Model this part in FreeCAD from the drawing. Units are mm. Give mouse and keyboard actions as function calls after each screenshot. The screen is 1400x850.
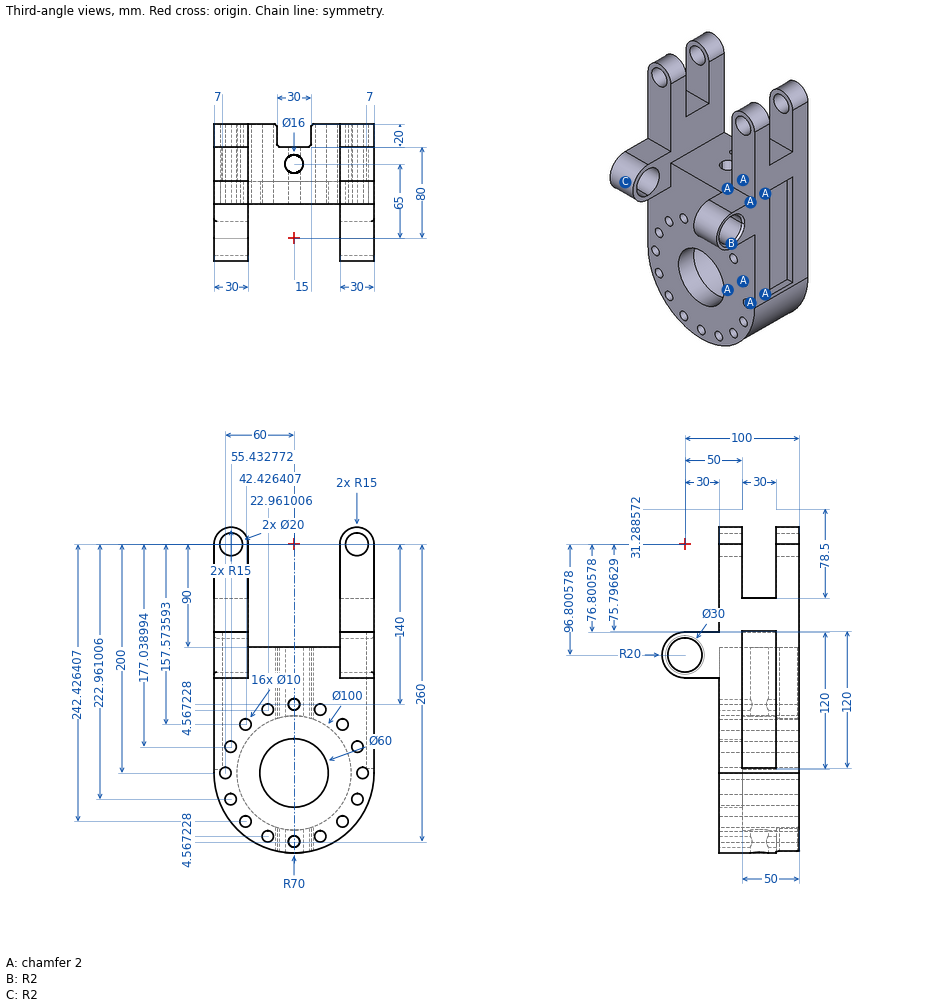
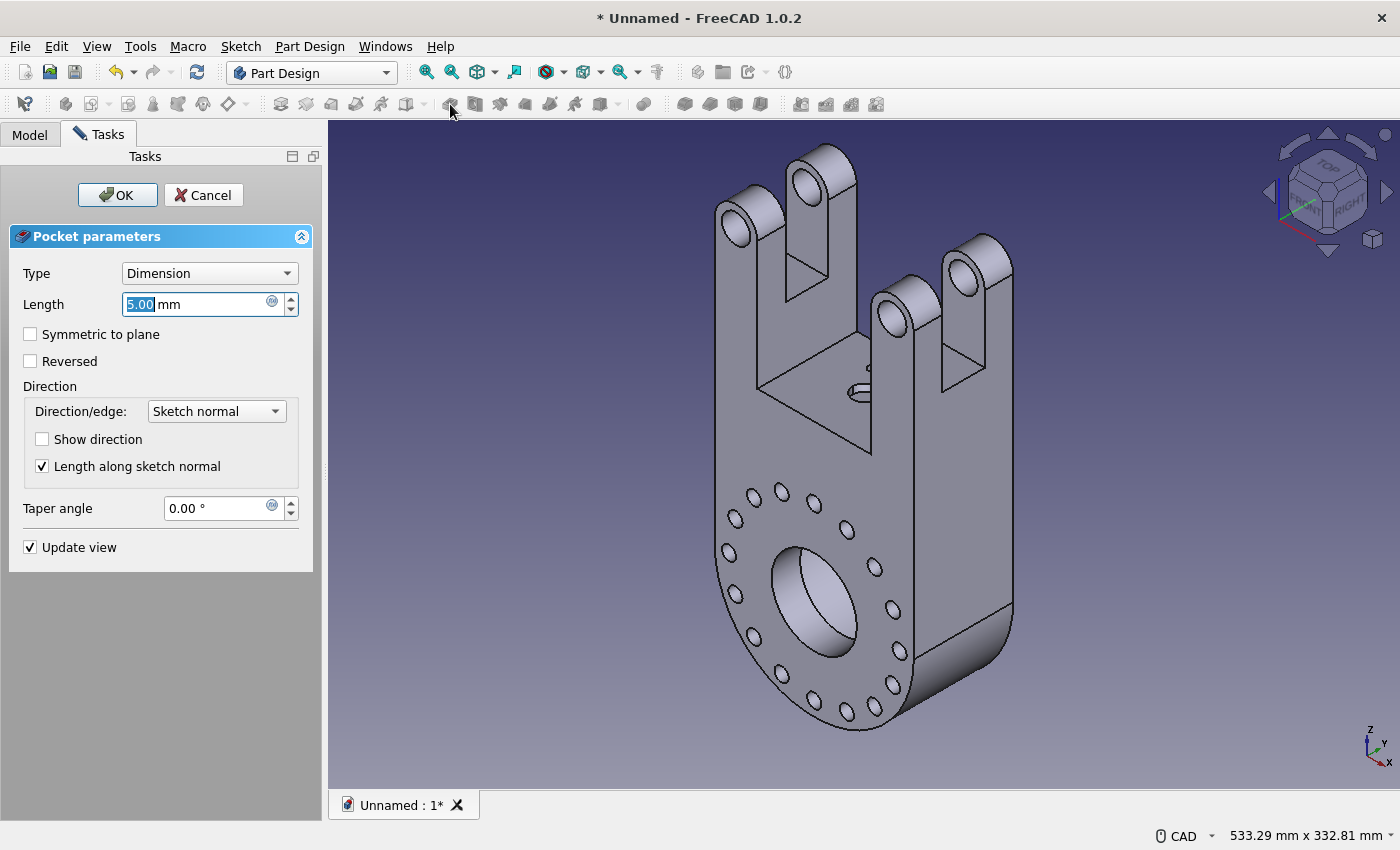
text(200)
key(Tab)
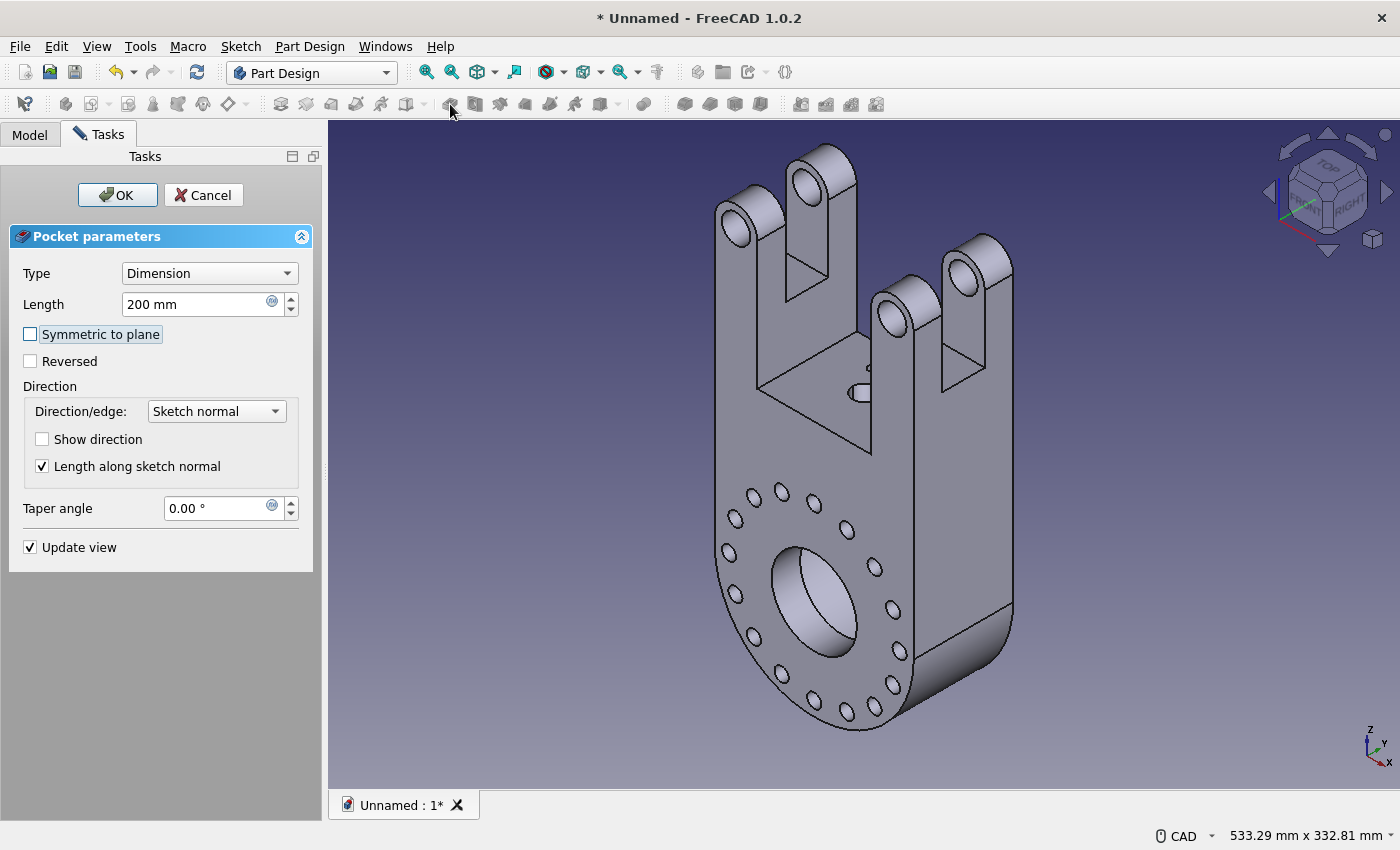
click(118, 195)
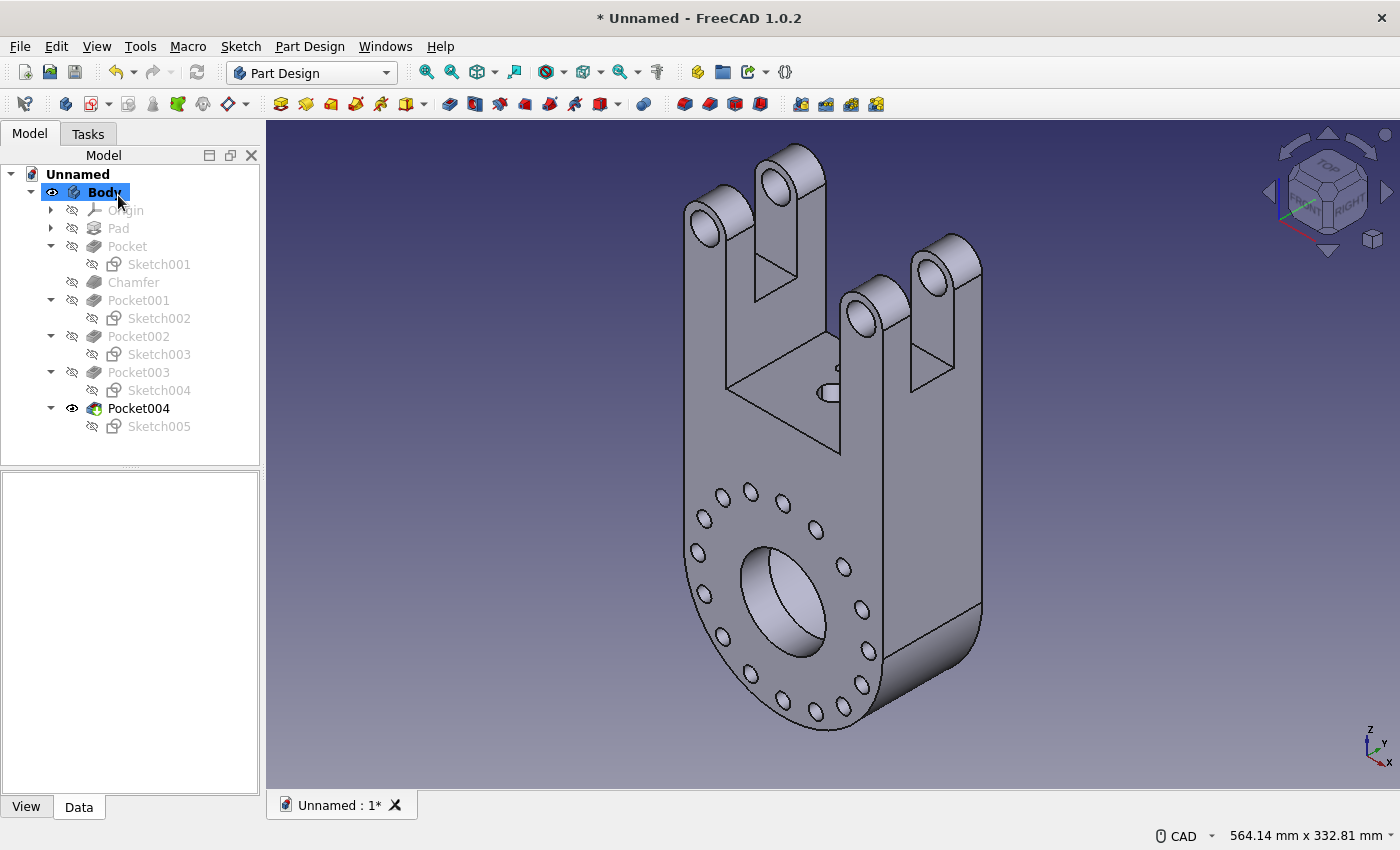
key(6)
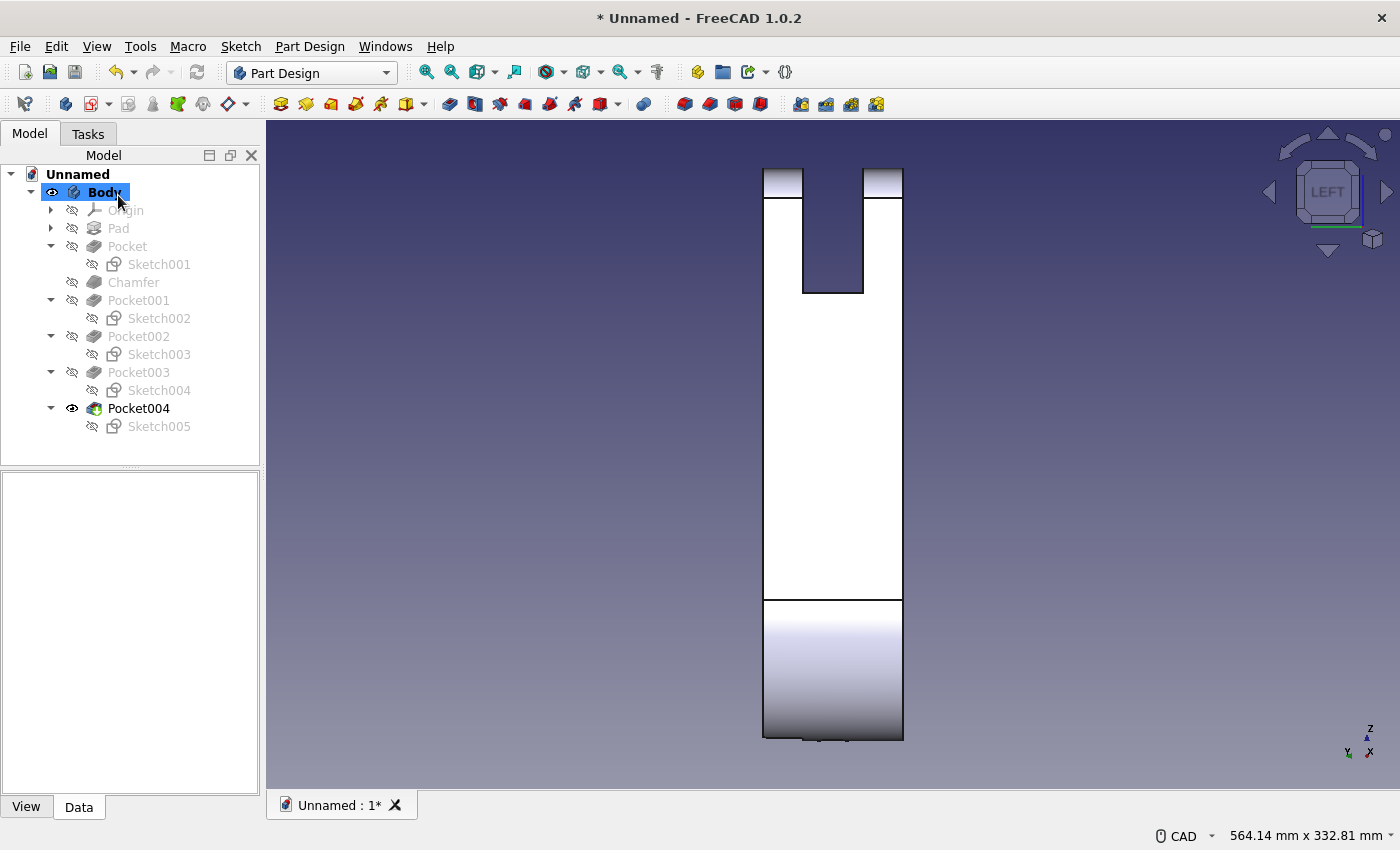
click(833, 513)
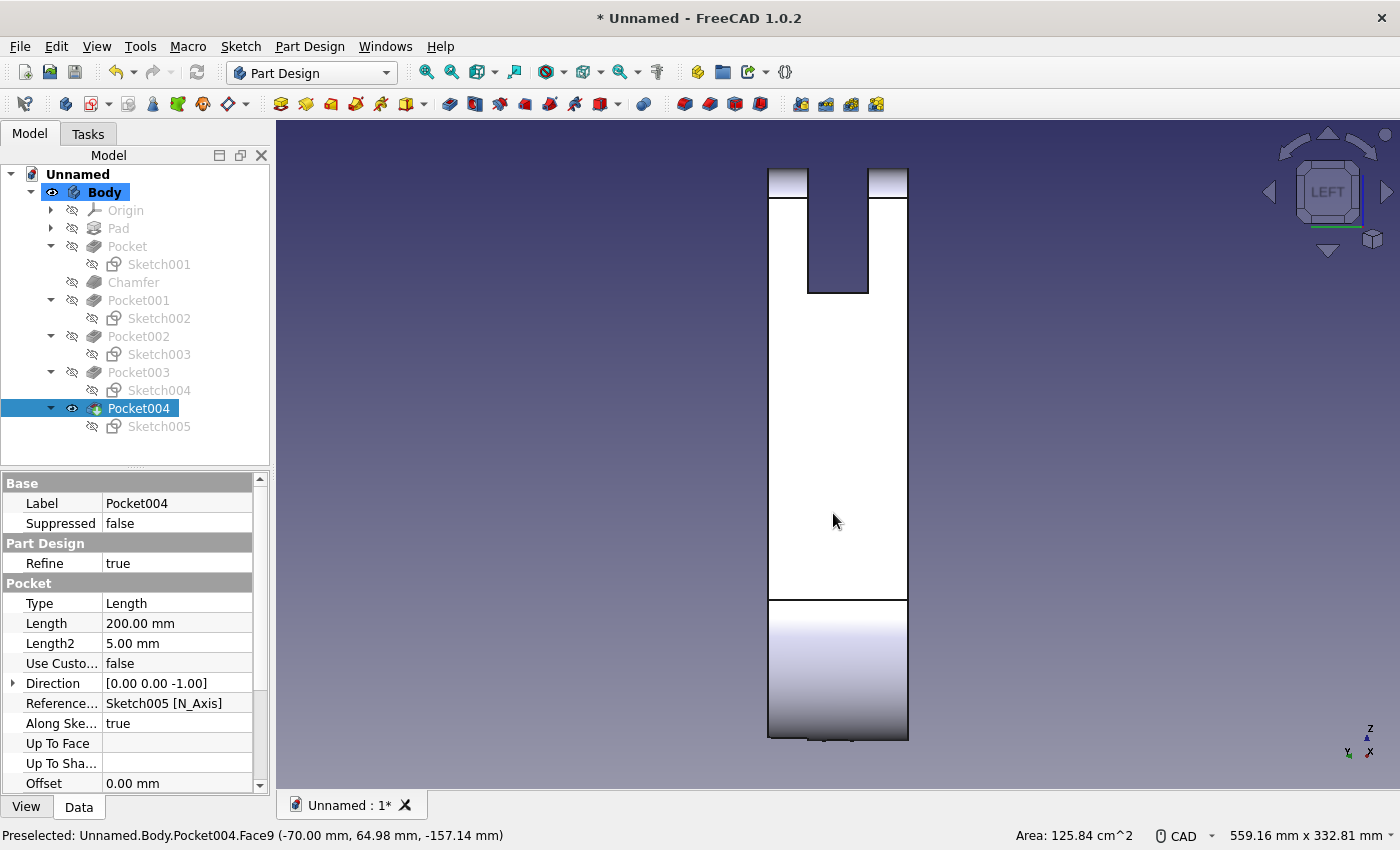
click(90, 104)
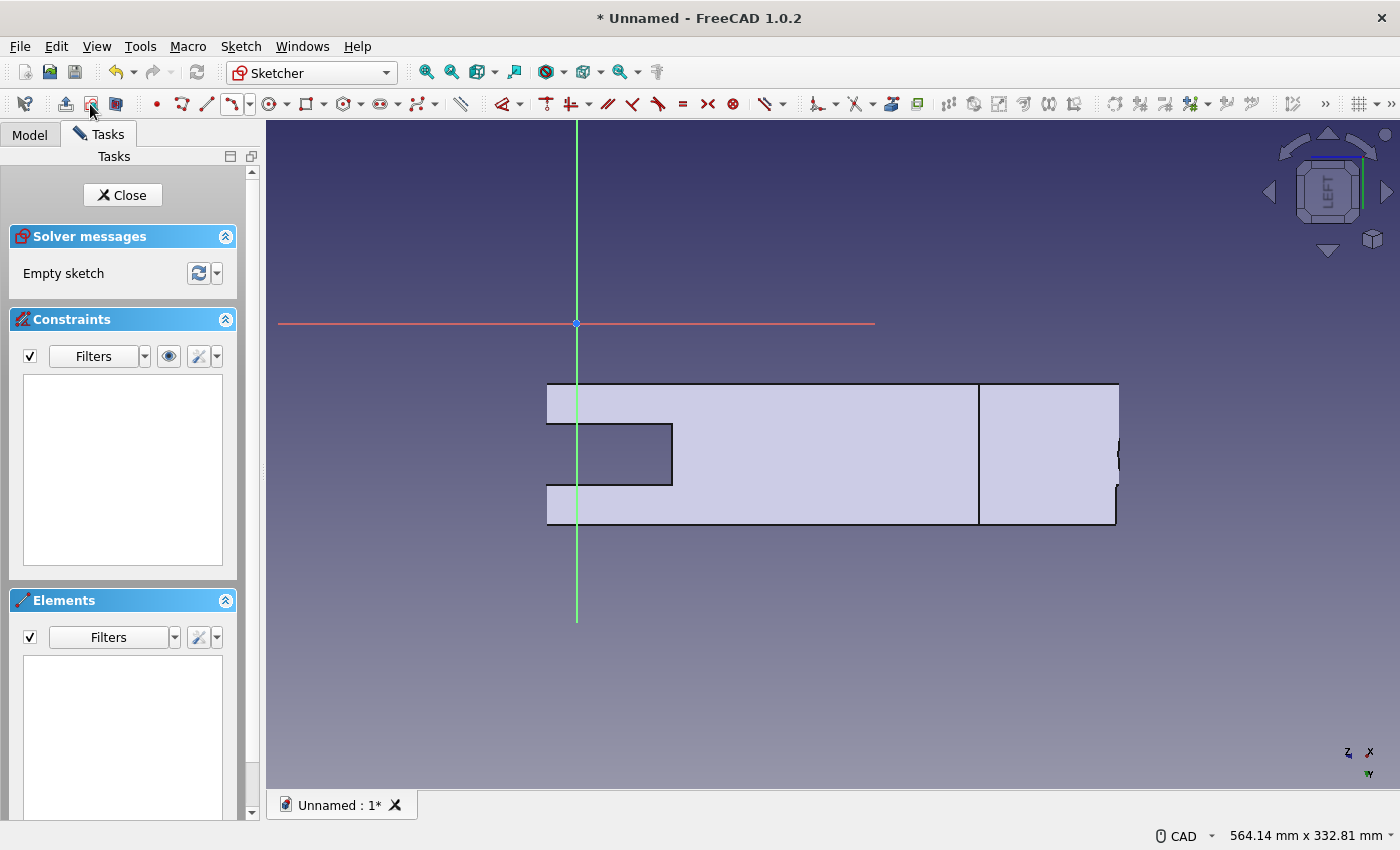
scroll(787, 343, up, 3)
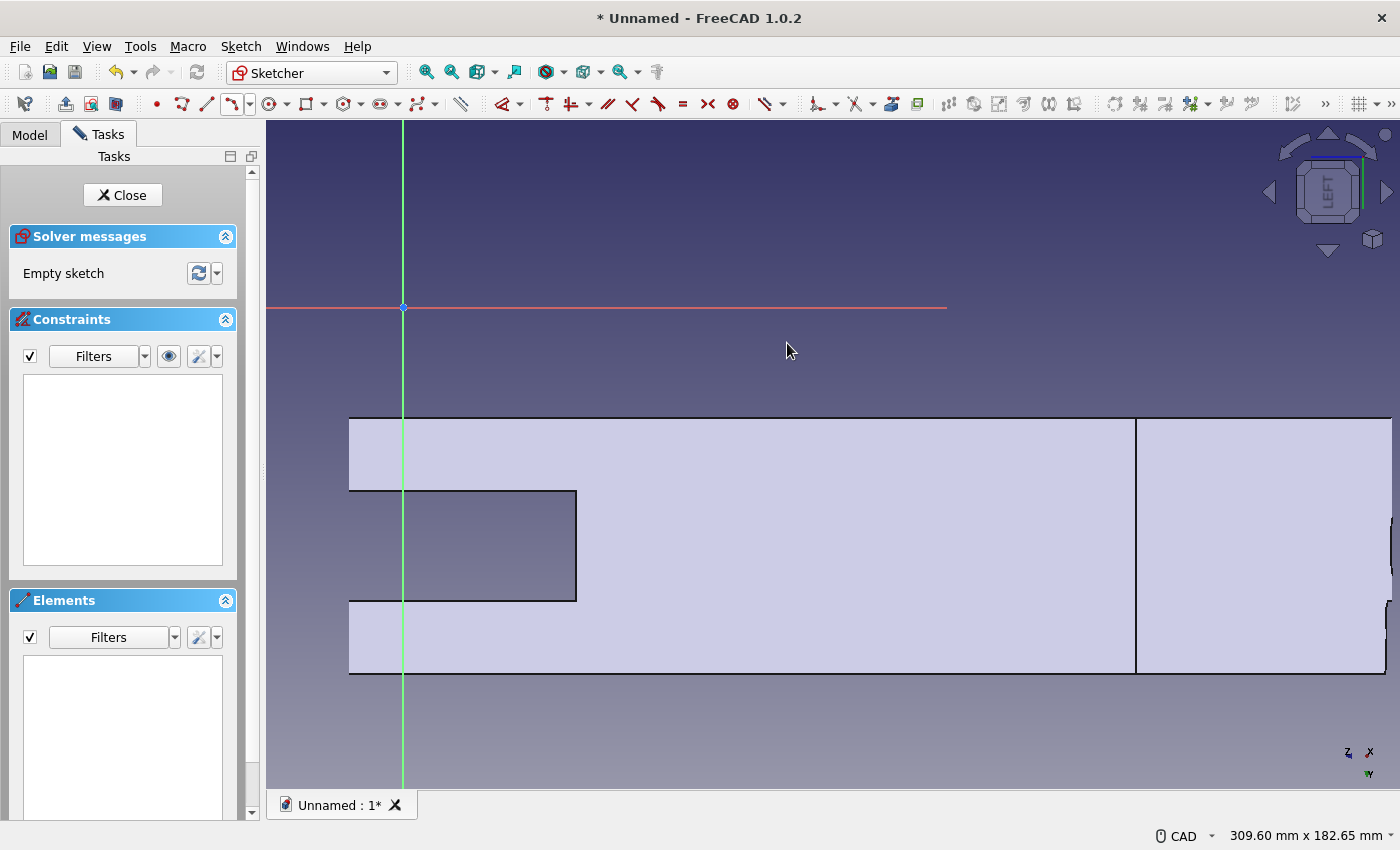
click(306, 104)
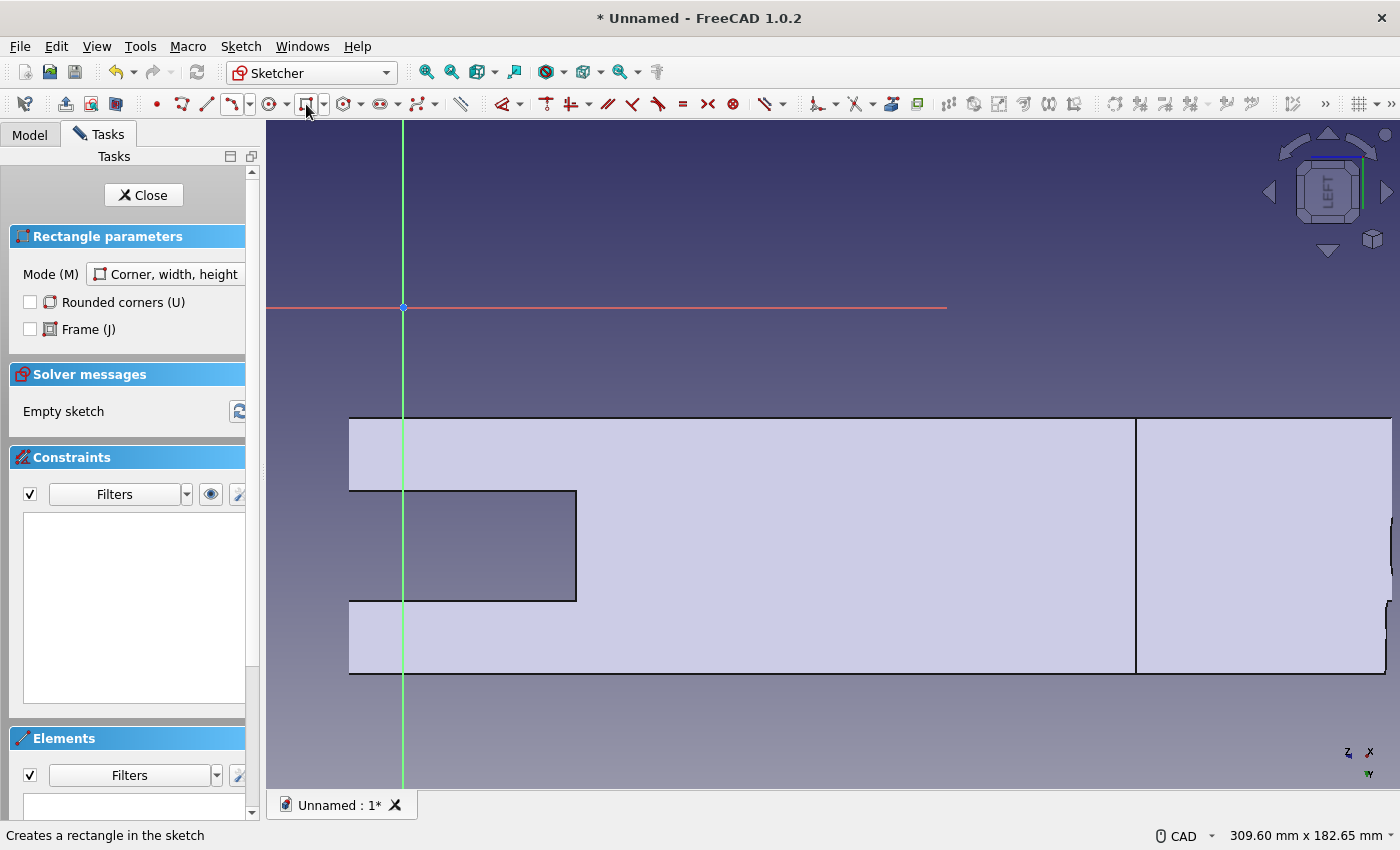
click(685, 491)
click(1124, 601)
key(Escape)